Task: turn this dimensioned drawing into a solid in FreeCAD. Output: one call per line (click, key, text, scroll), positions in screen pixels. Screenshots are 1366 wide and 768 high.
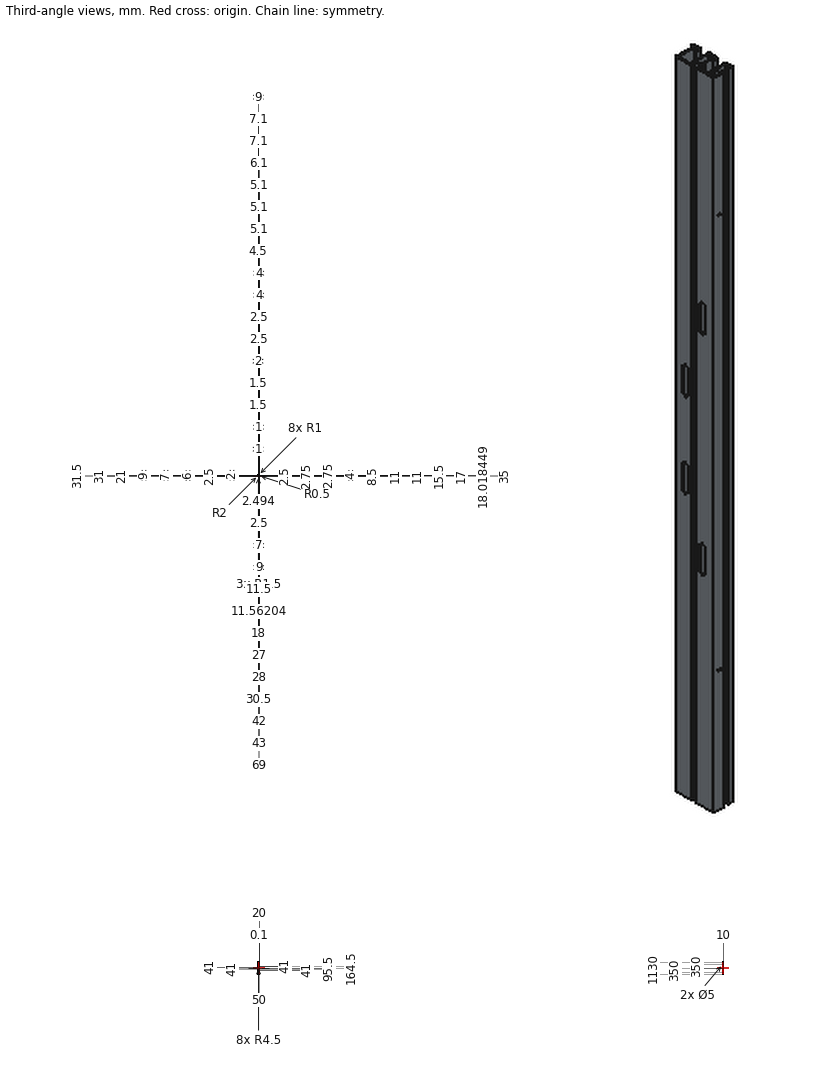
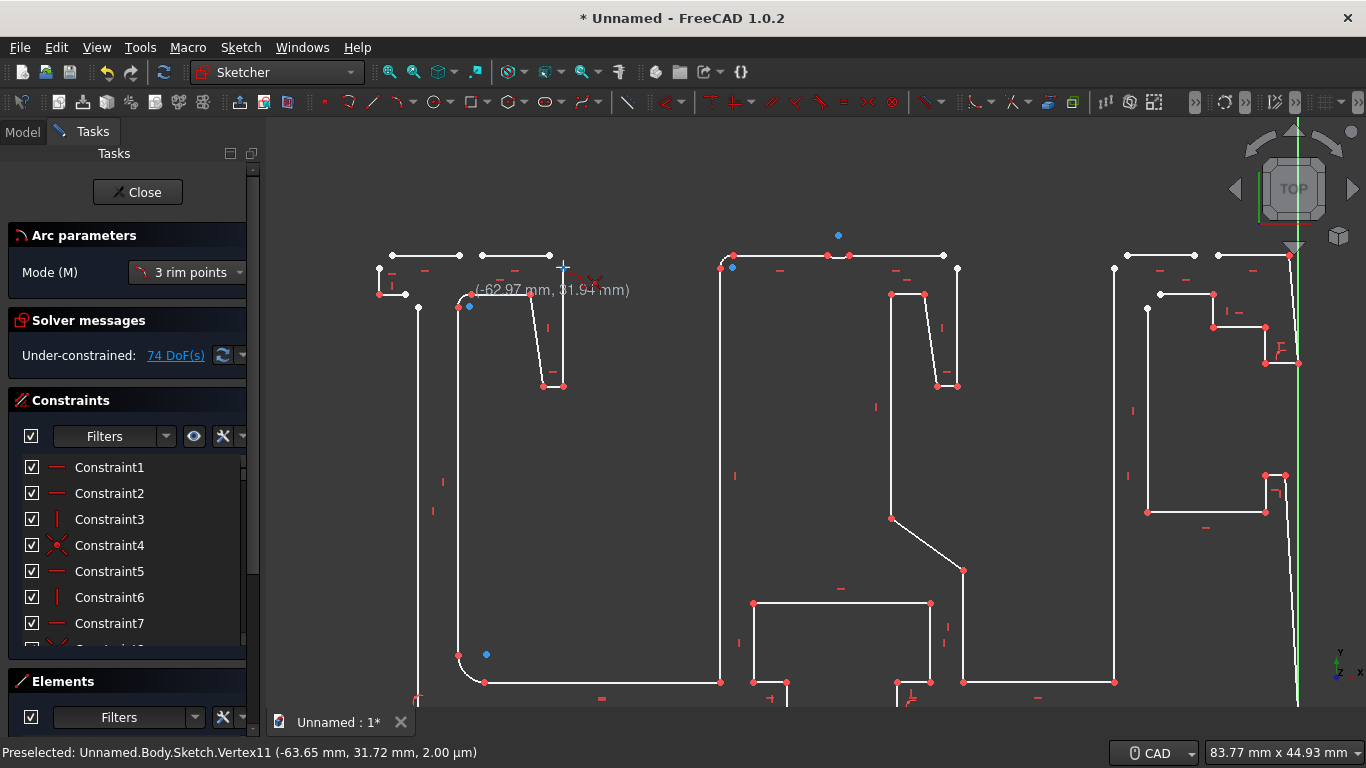
click(563, 269)
click(549, 256)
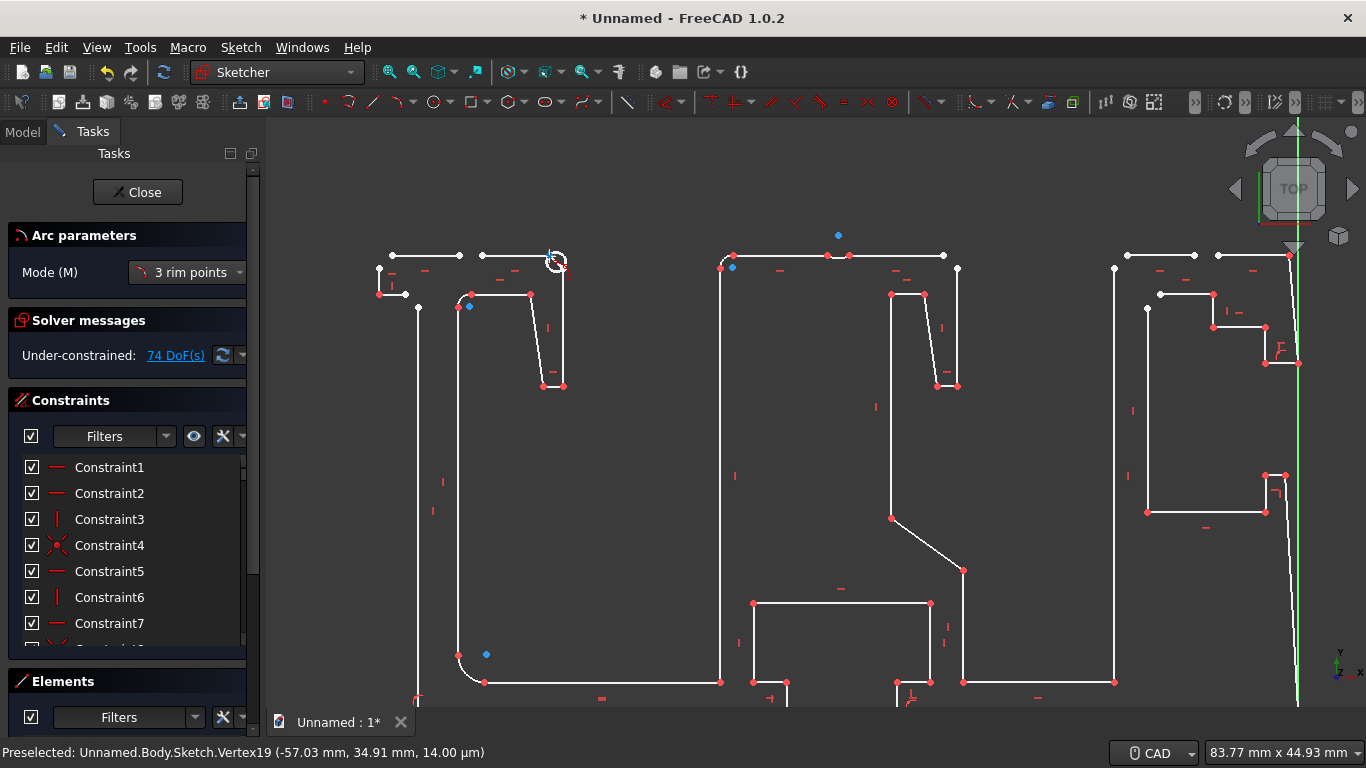
scroll(559, 258, up, 8)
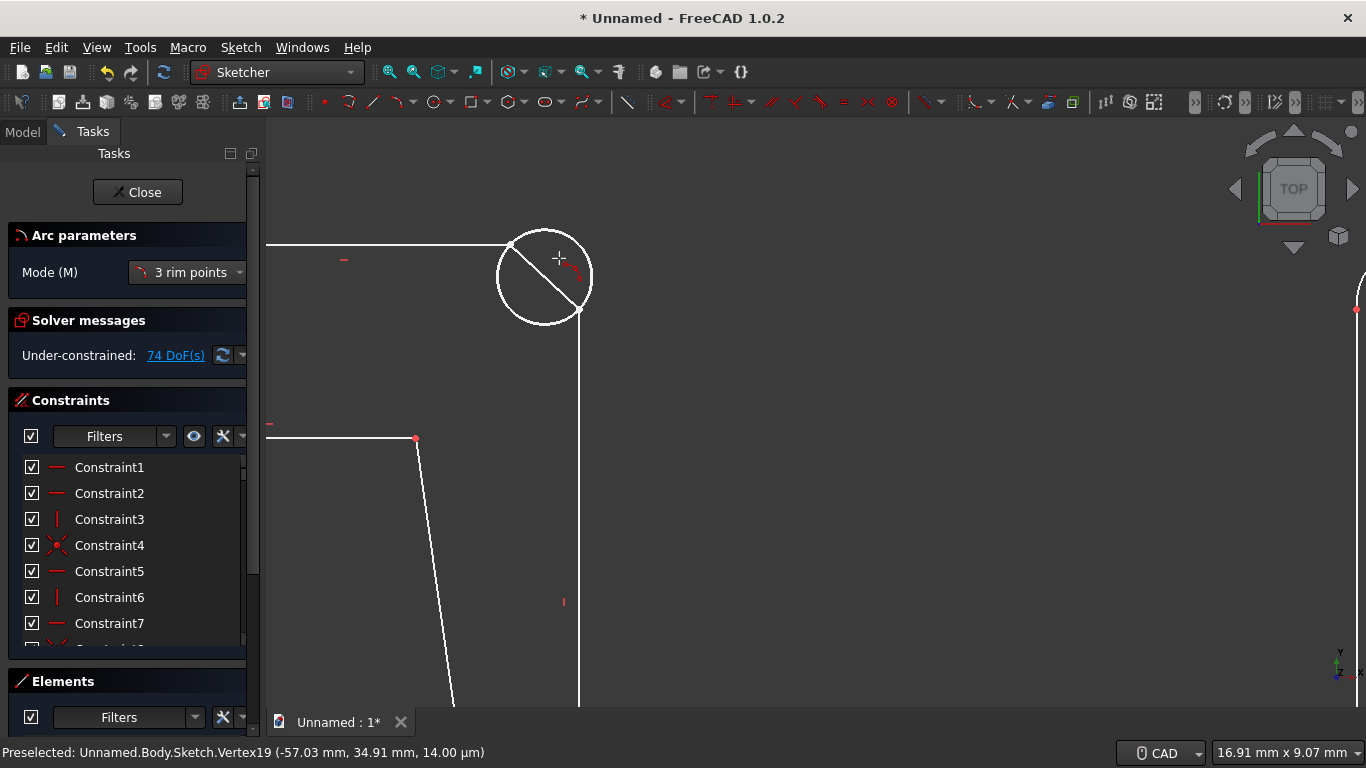
click(558, 258)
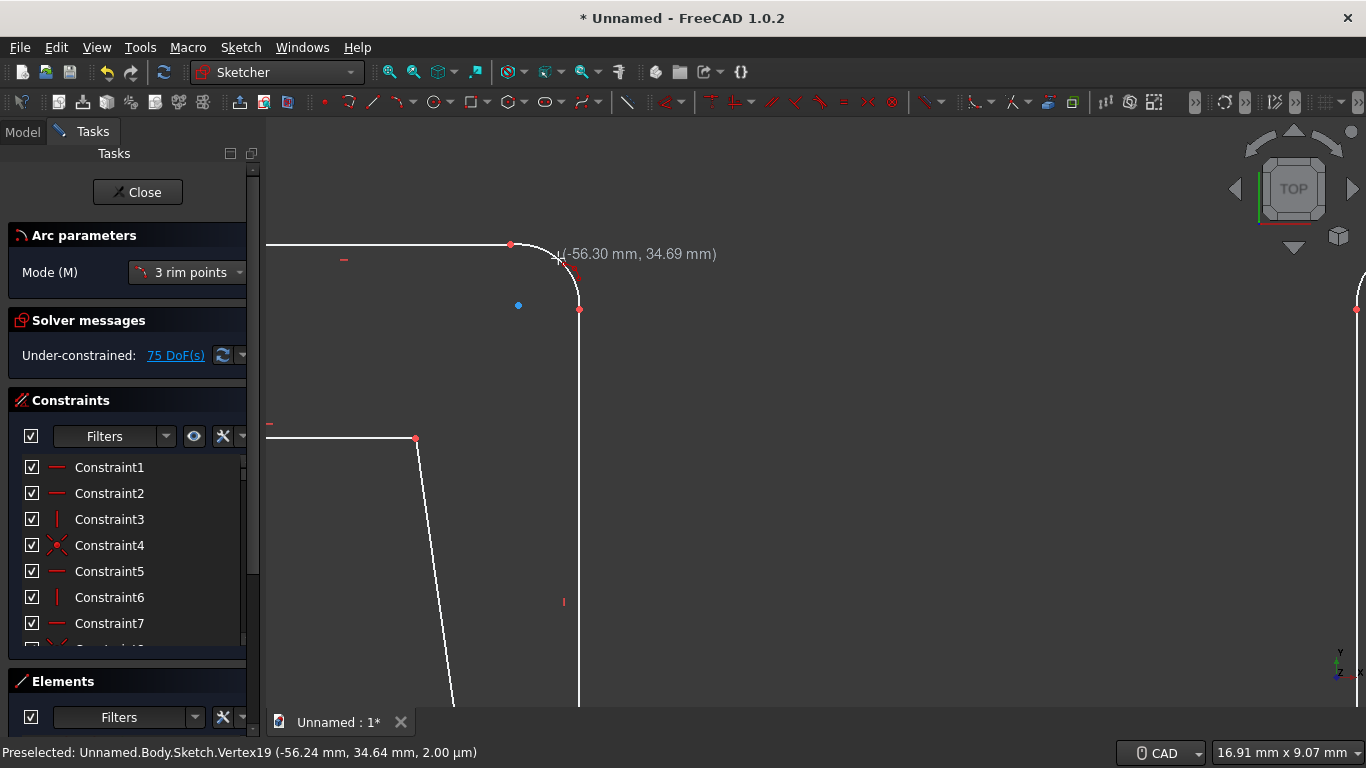
scroll(560, 261, down, 10)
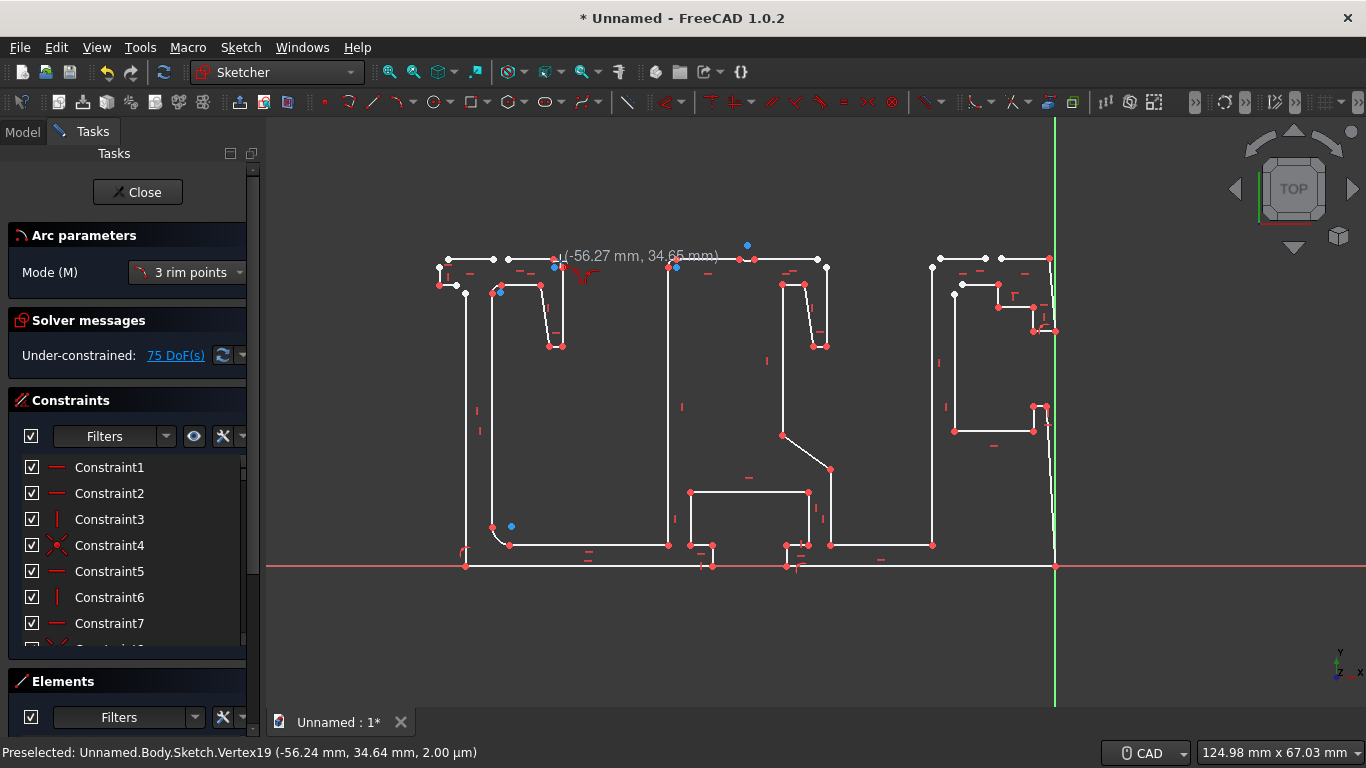
click(509, 259)
click(493, 259)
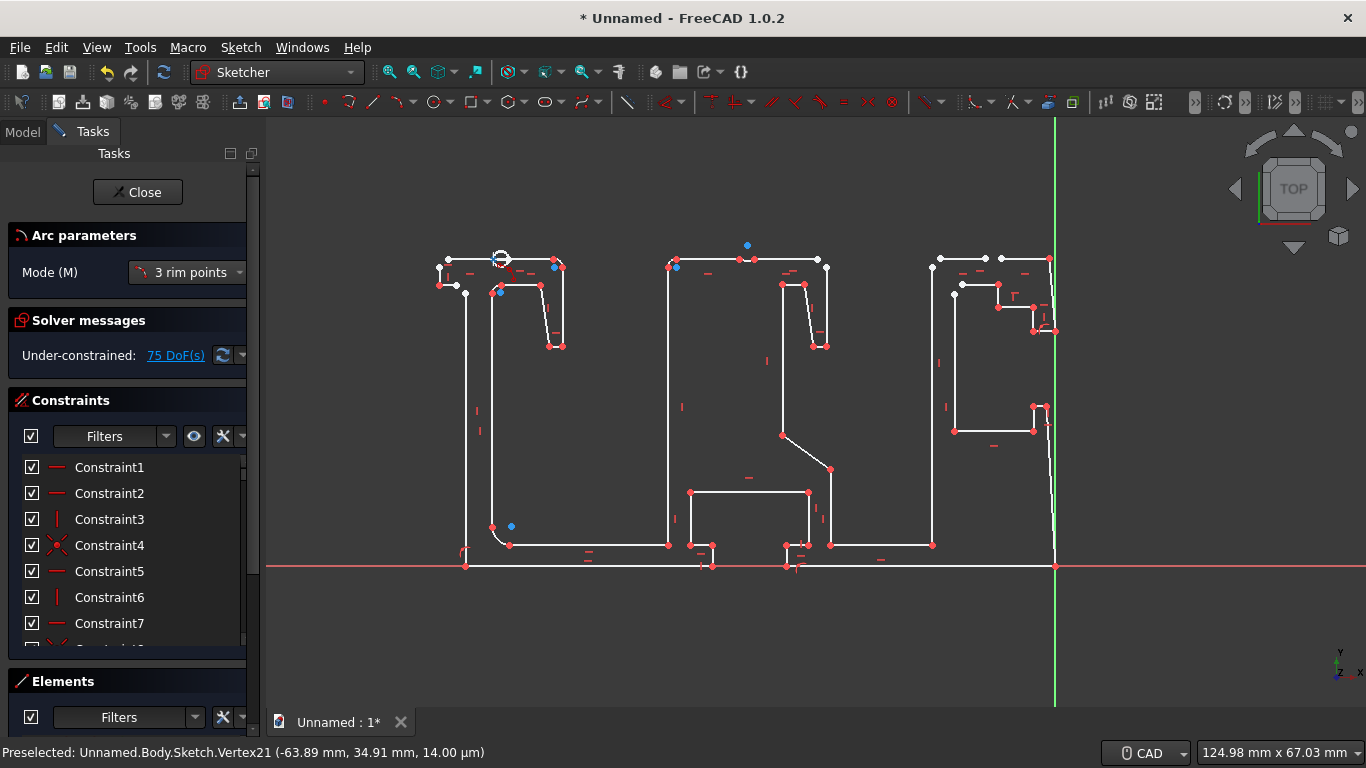
scroll(501, 261, up, 9)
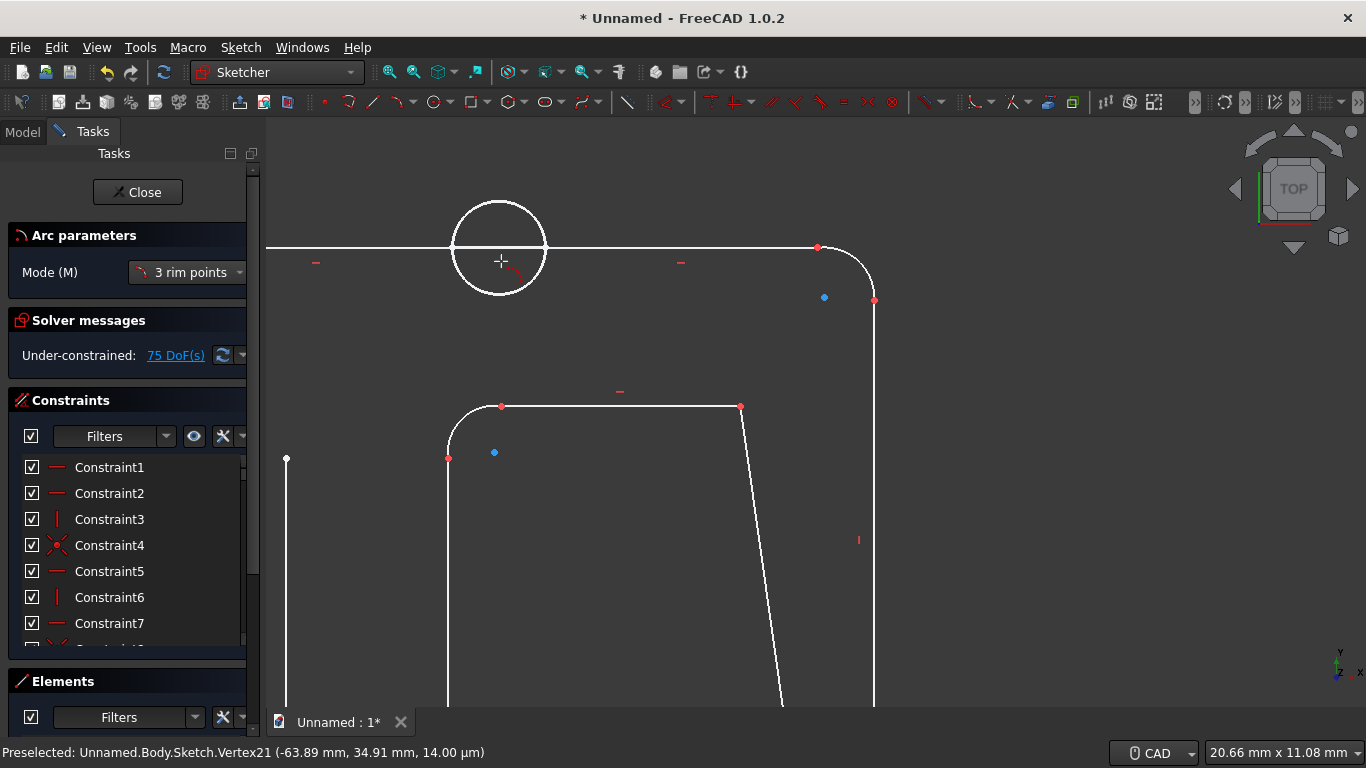
click(500, 259)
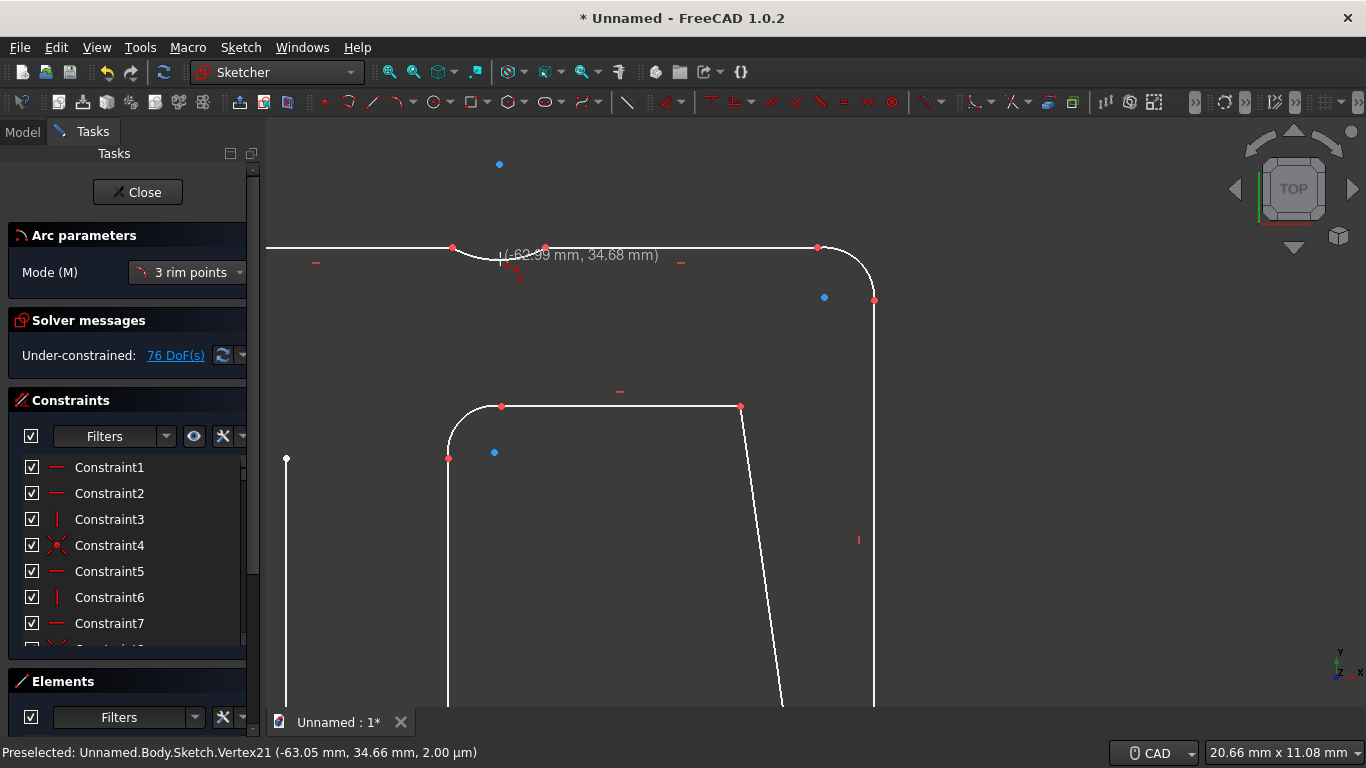
scroll(501, 261, down, 9)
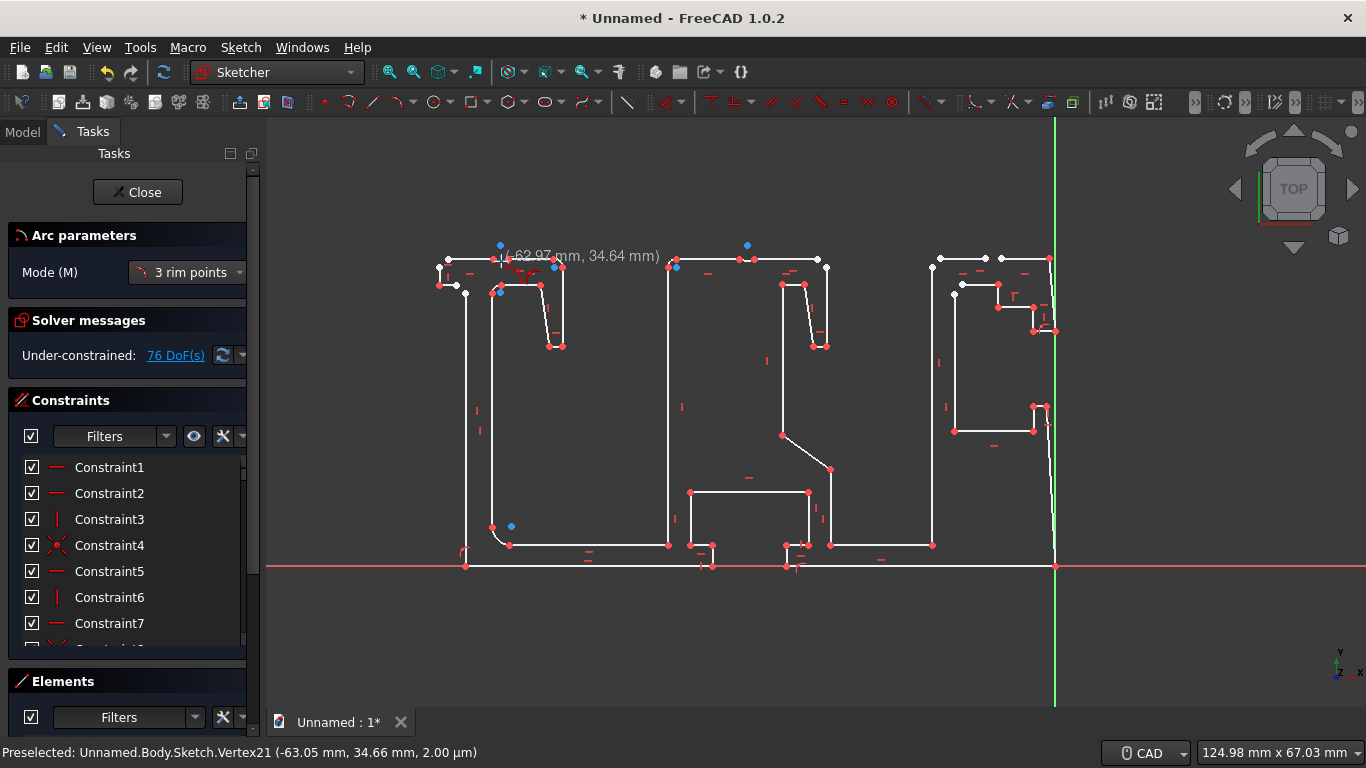
scroll(448, 258, up, 2)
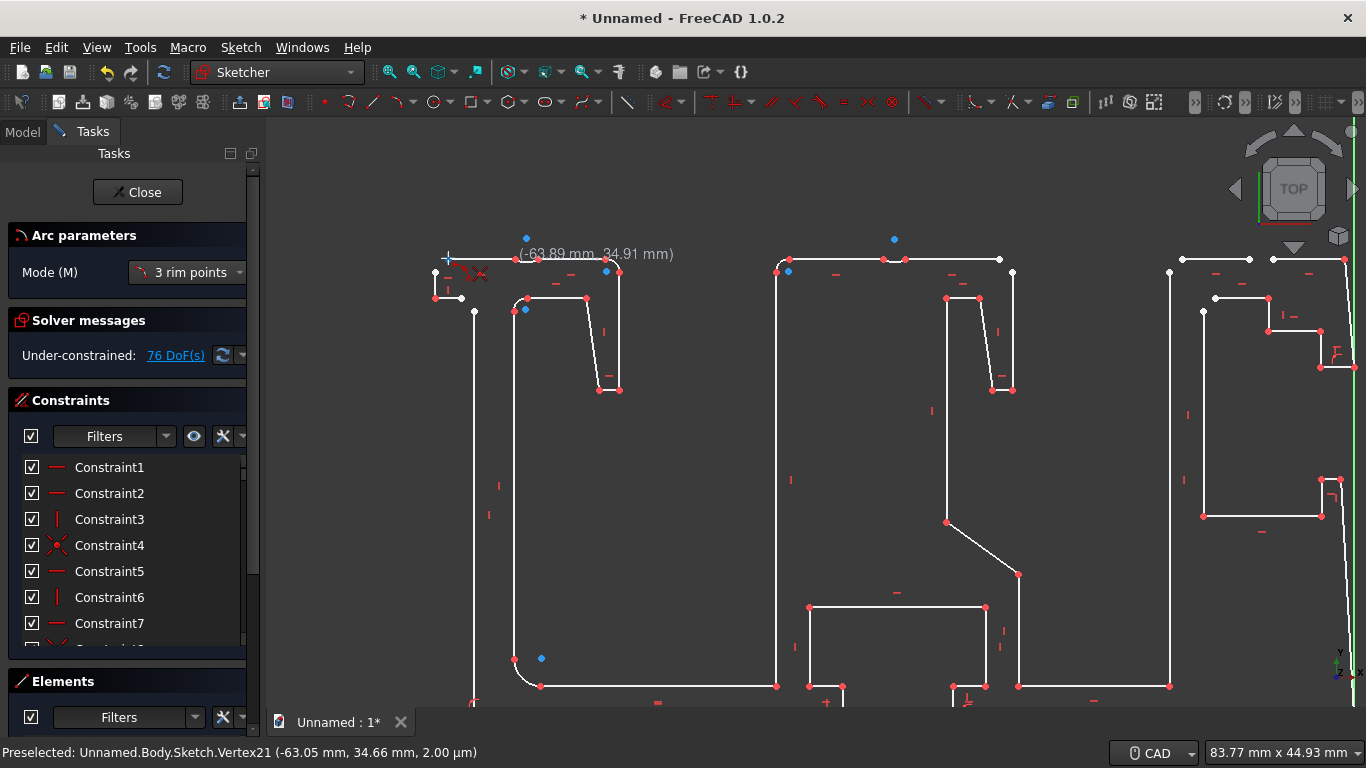
click(448, 259)
click(435, 272)